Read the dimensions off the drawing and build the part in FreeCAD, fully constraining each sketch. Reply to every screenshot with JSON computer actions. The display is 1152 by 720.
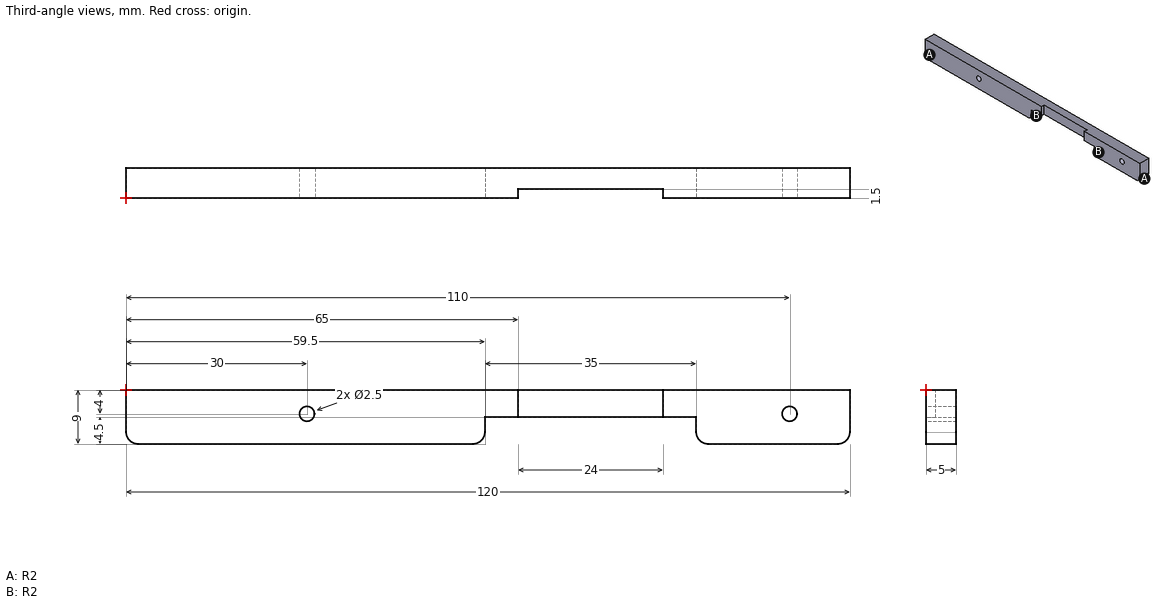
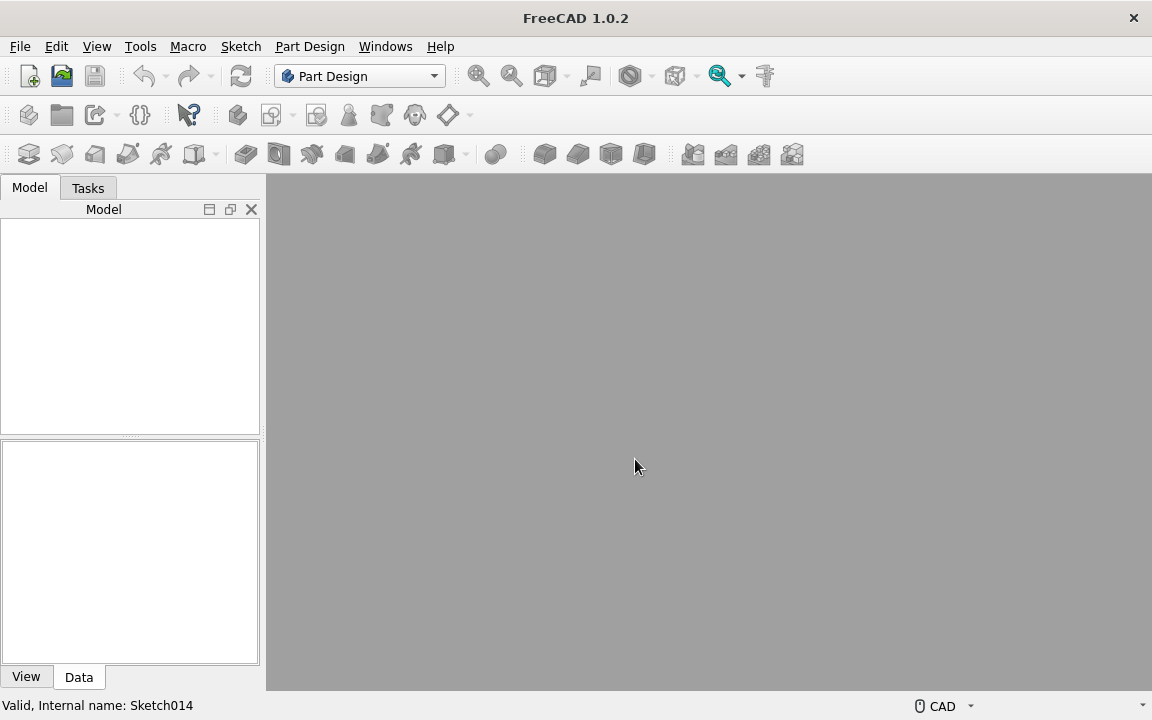
{"action": "key", "text": "ctrl+n"}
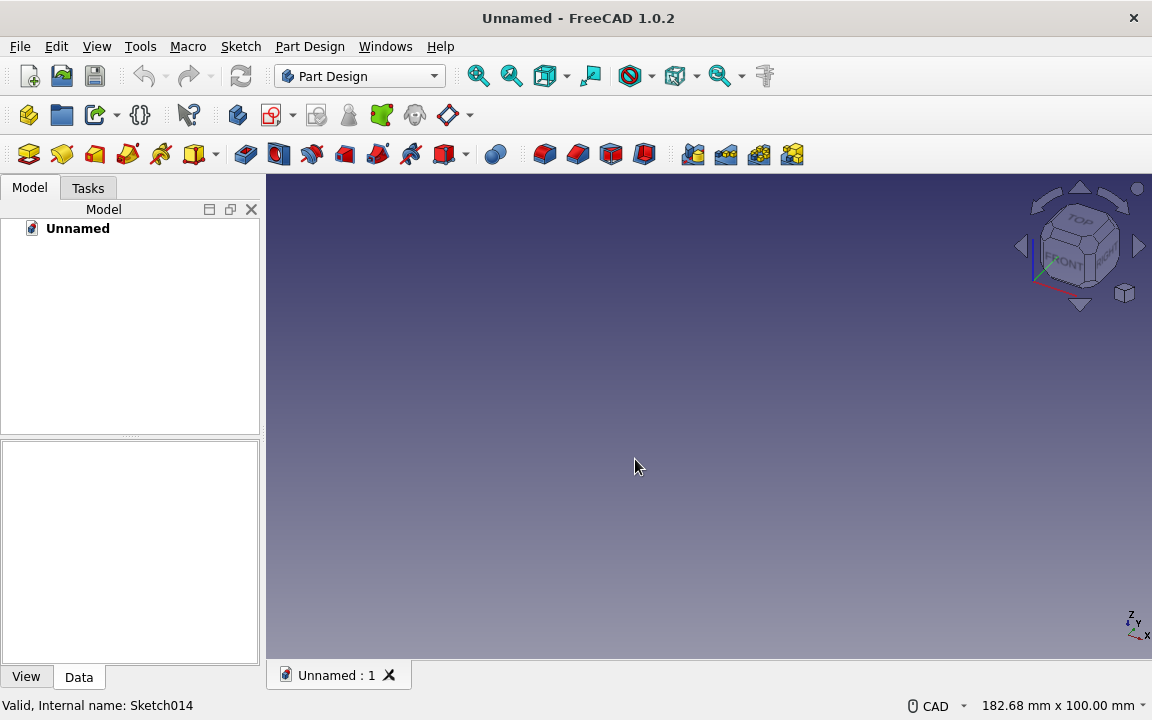
{"action": "left_click", "coordinate": [270, 116]}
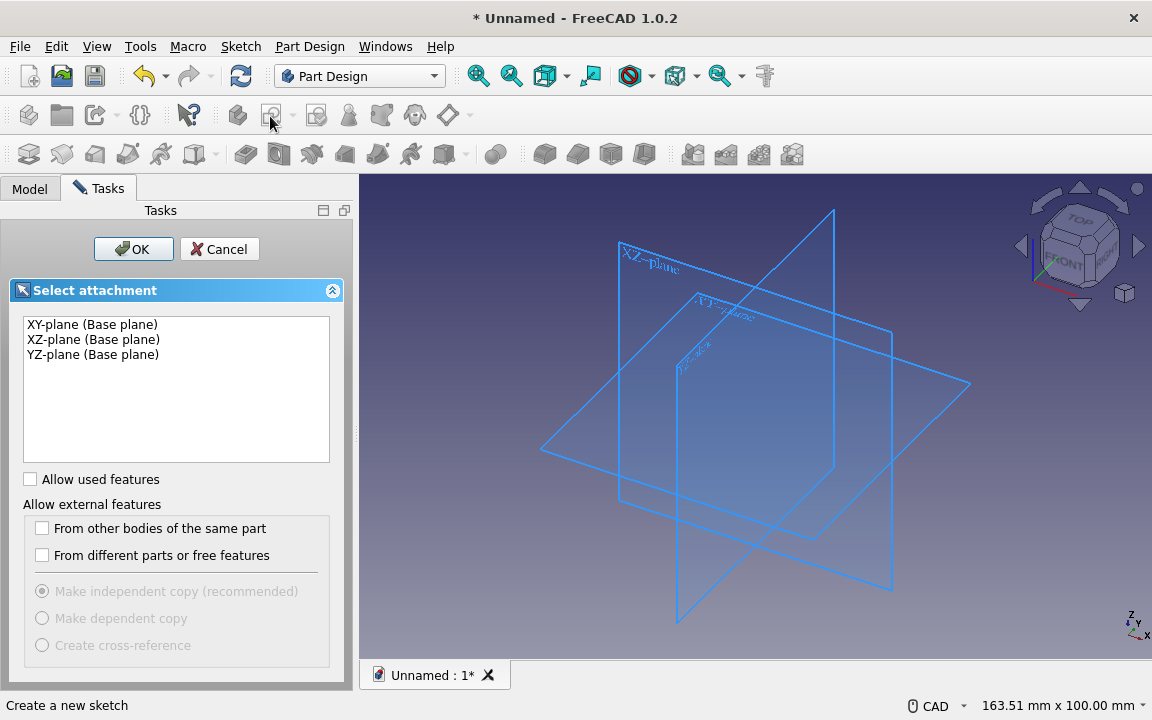
{"action": "left_click", "coordinate": [84, 340]}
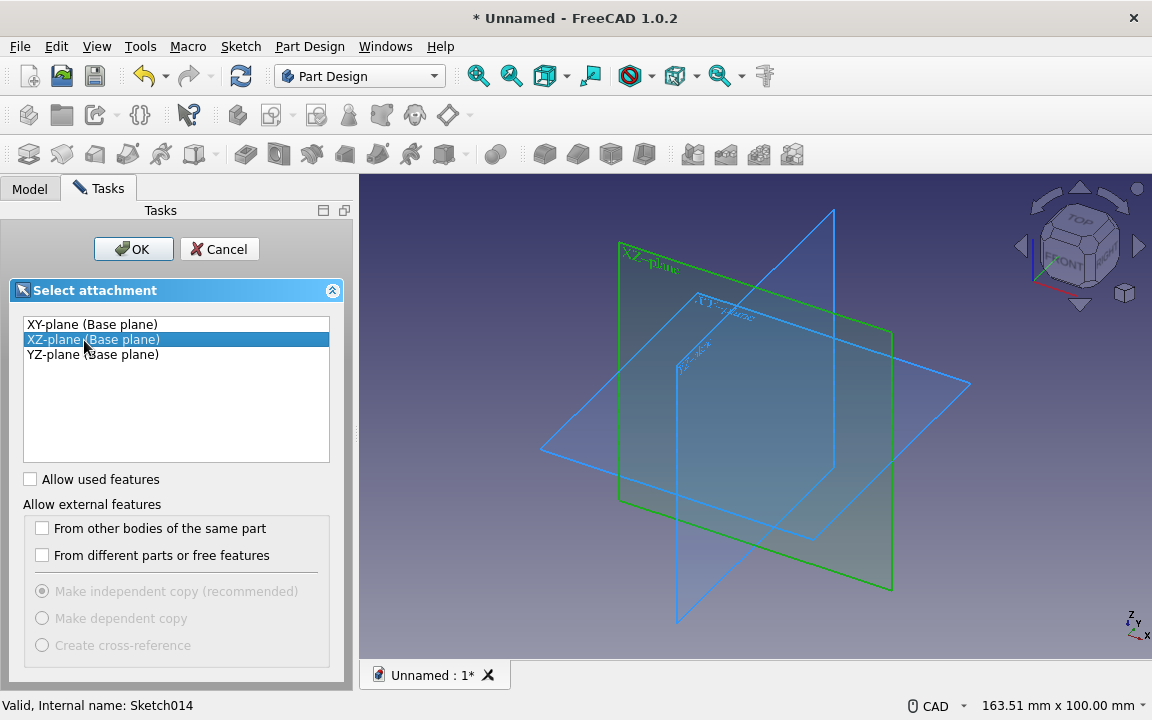
{"action": "left_click", "coordinate": [134, 249]}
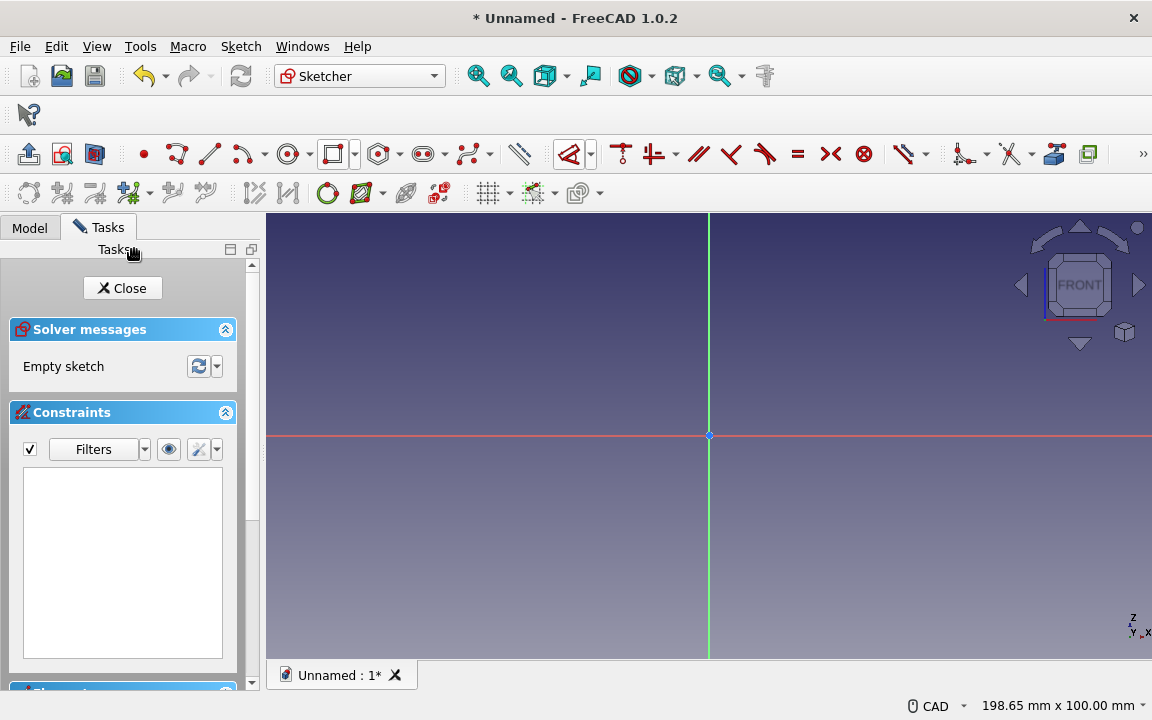
{"action": "scroll", "coordinate": [294, 395], "scroll_direction": "down", "scroll_amount": 2}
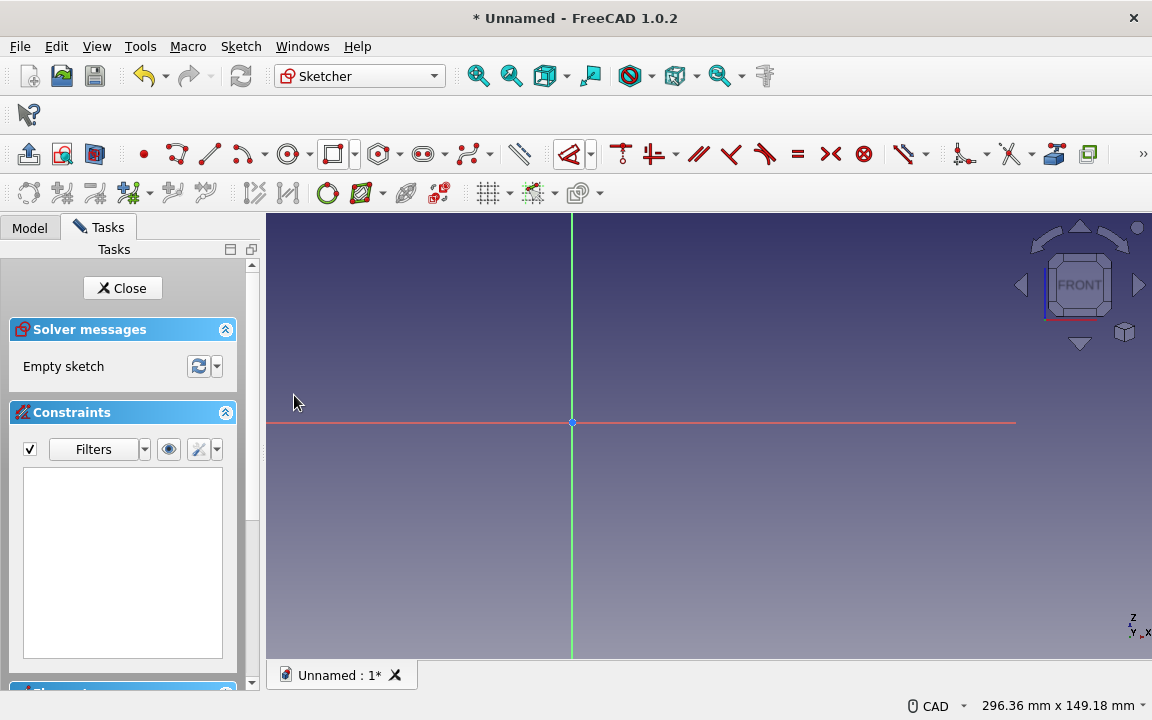
{"action": "scroll", "coordinate": [977, 436], "scroll_direction": "up", "scroll_amount": 2}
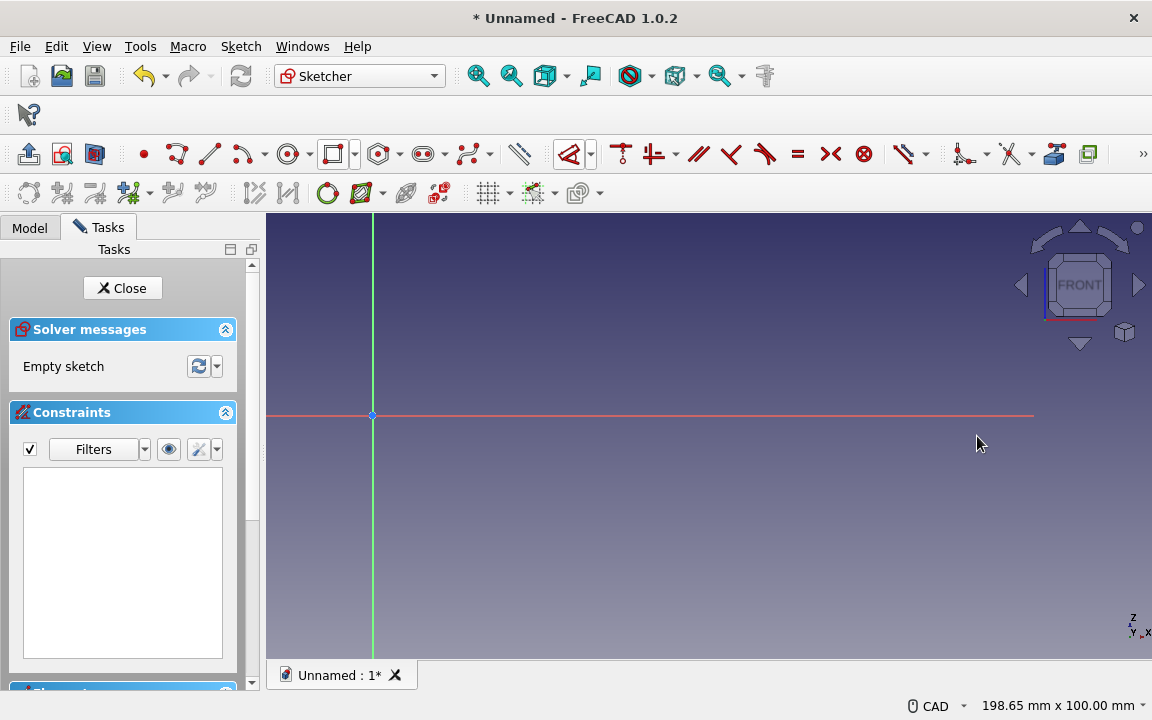
{"action": "left_click", "coordinate": [332, 154]}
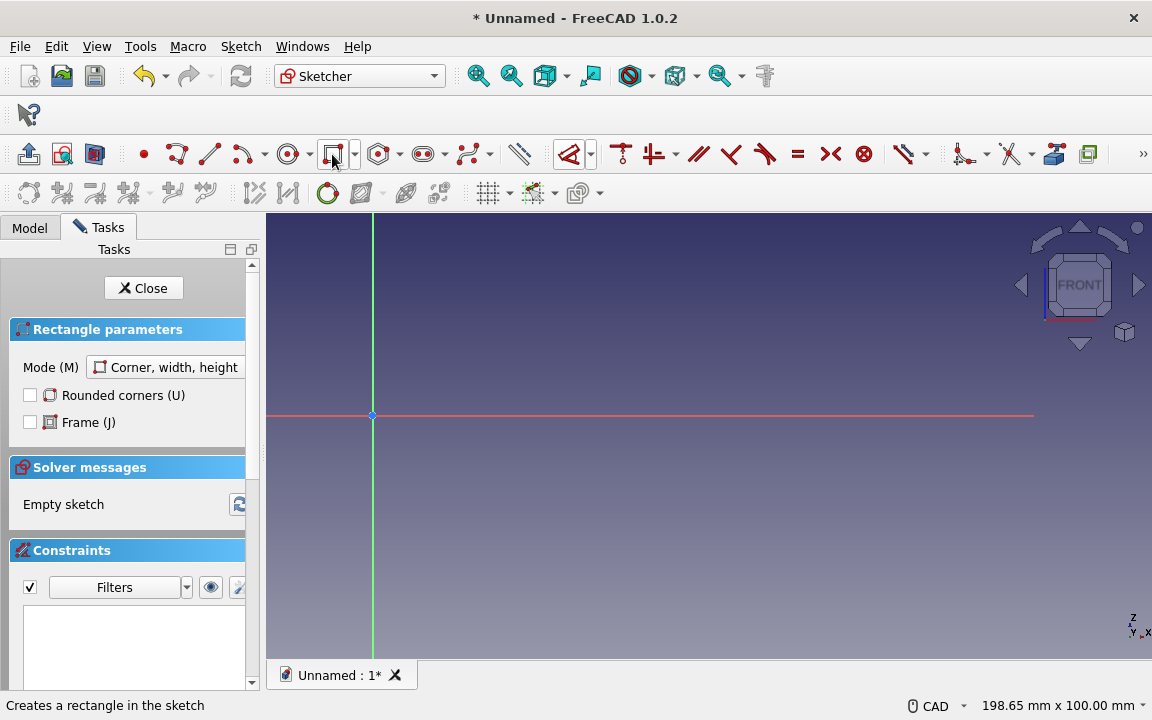
{"action": "left_click", "coordinate": [373, 416]}
{"action": "left_click", "coordinate": [908, 456]}
{"action": "key", "text": "Escape"}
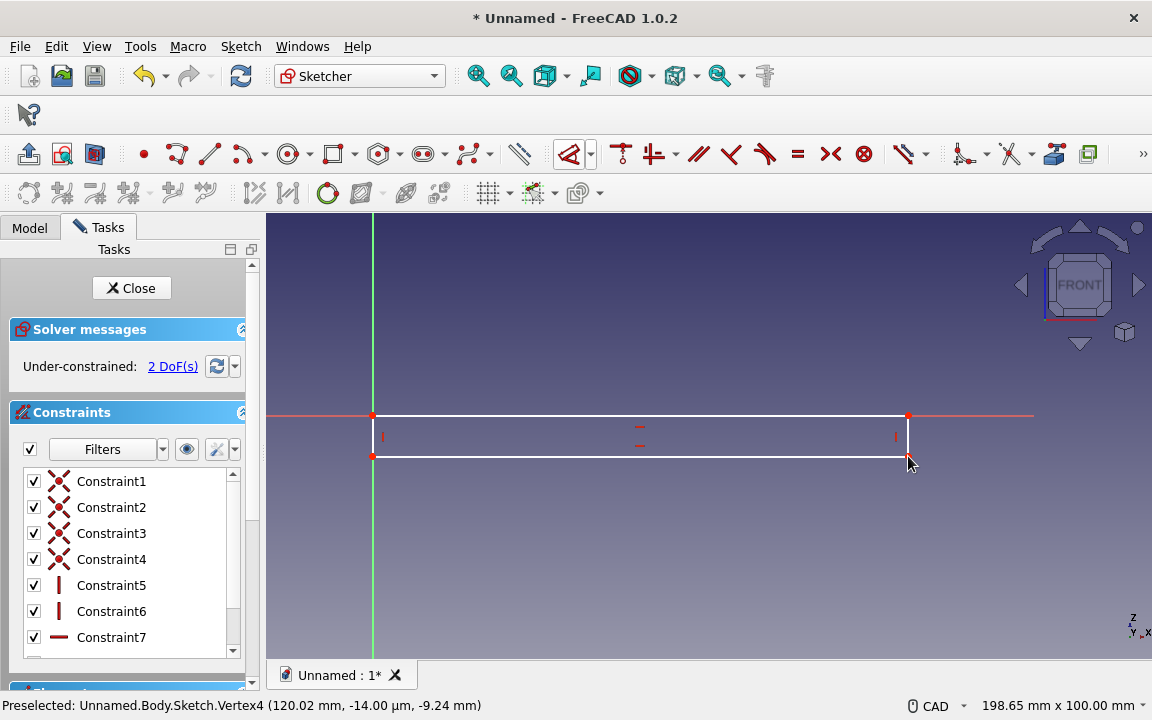
{"action": "key", "text": "d"}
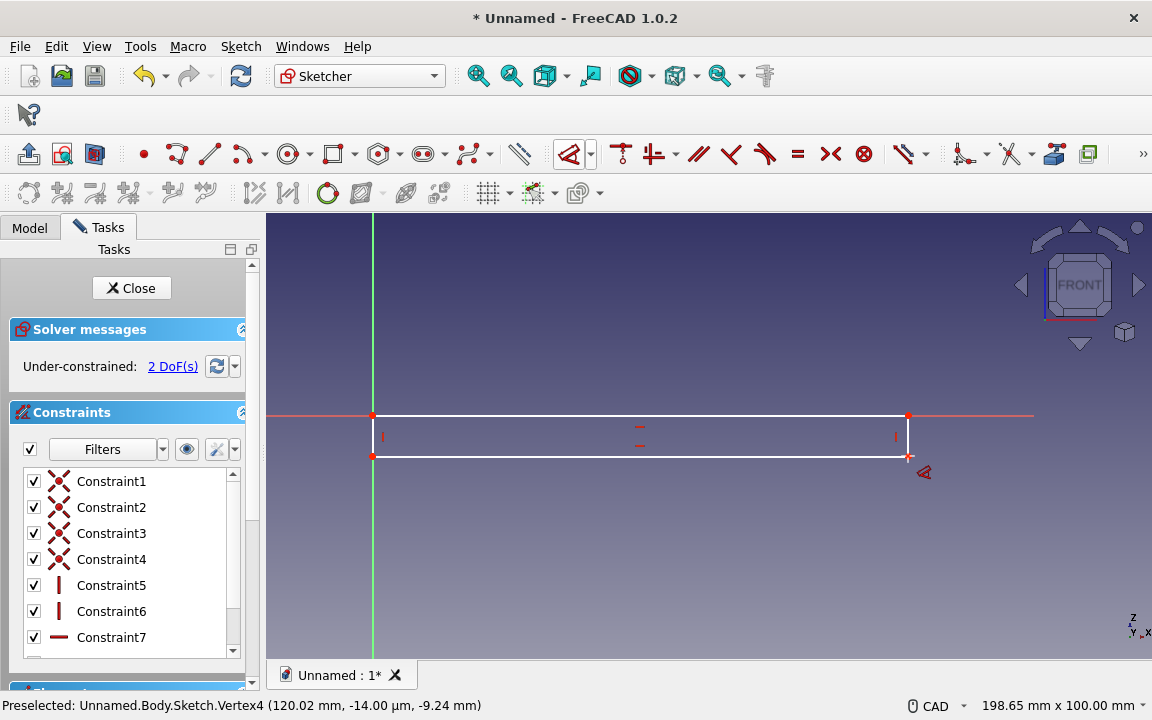
{"action": "left_click", "coordinate": [373, 428]}
{"action": "left_click", "coordinate": [339, 436]}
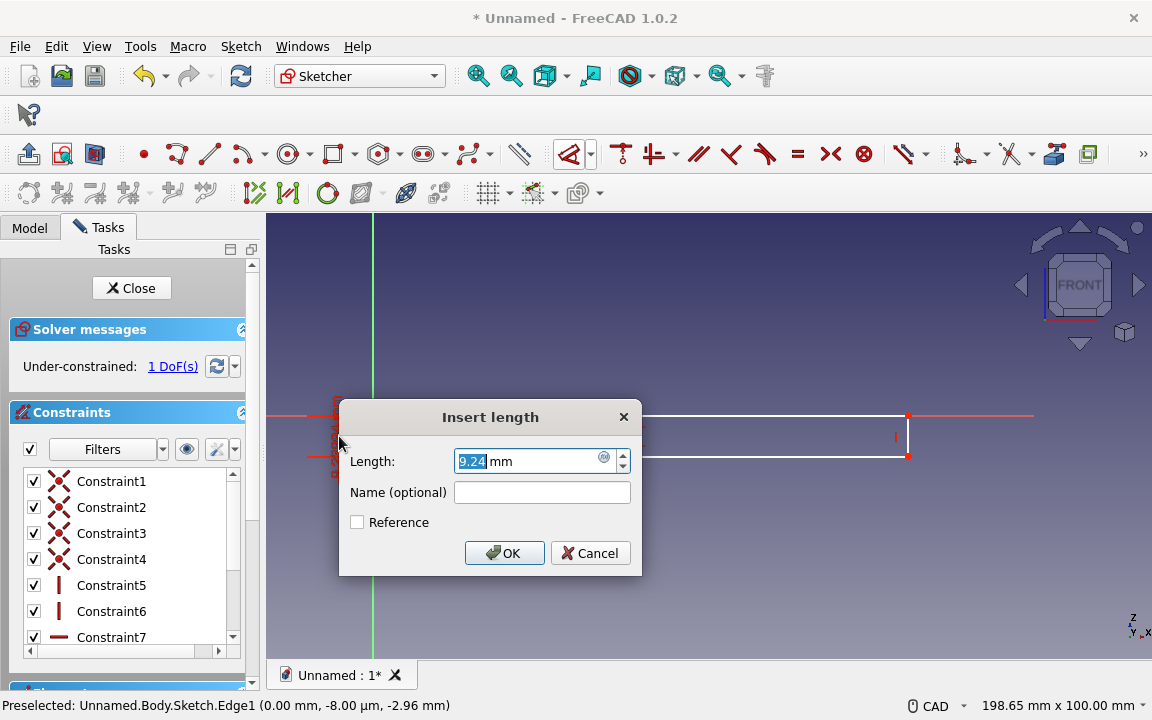
{"action": "type", "text": "9"}
{"action": "key", "text": "Return"}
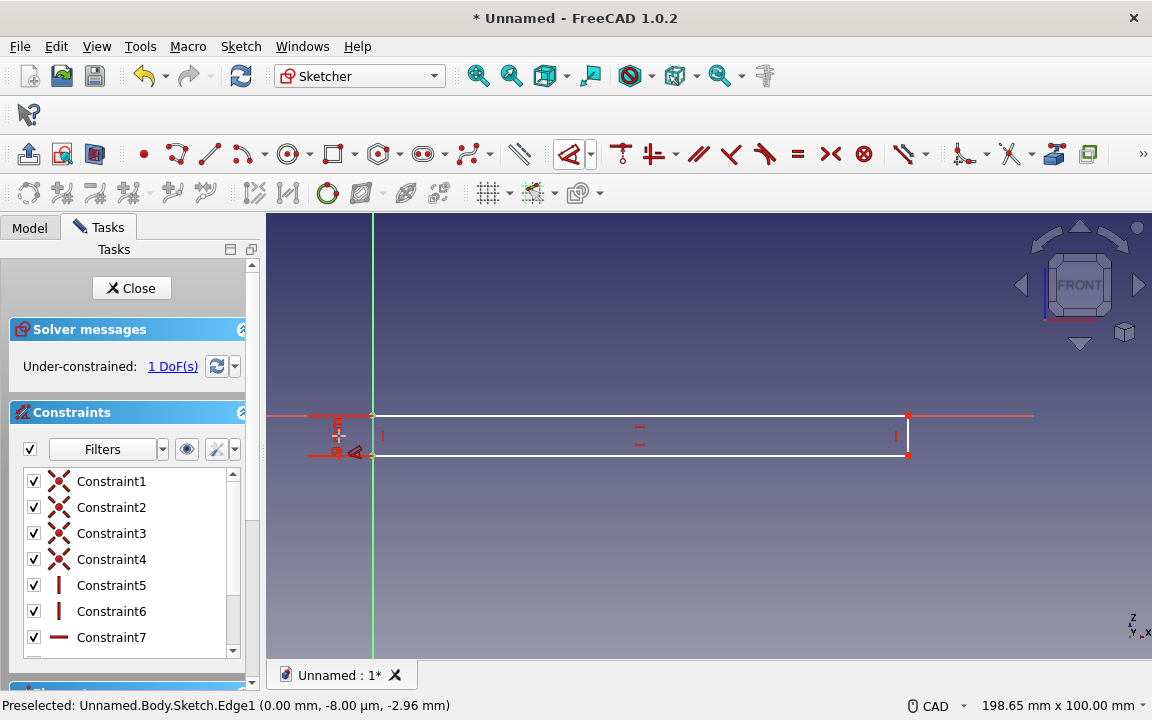
{"action": "left_click", "coordinate": [533, 456]}
{"action": "left_click", "coordinate": [640, 490]}